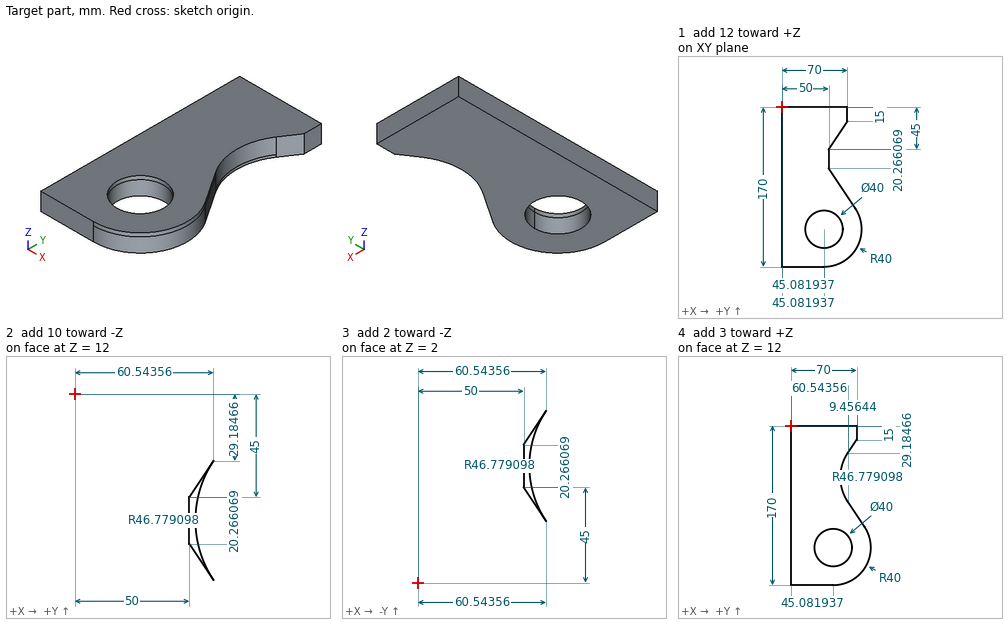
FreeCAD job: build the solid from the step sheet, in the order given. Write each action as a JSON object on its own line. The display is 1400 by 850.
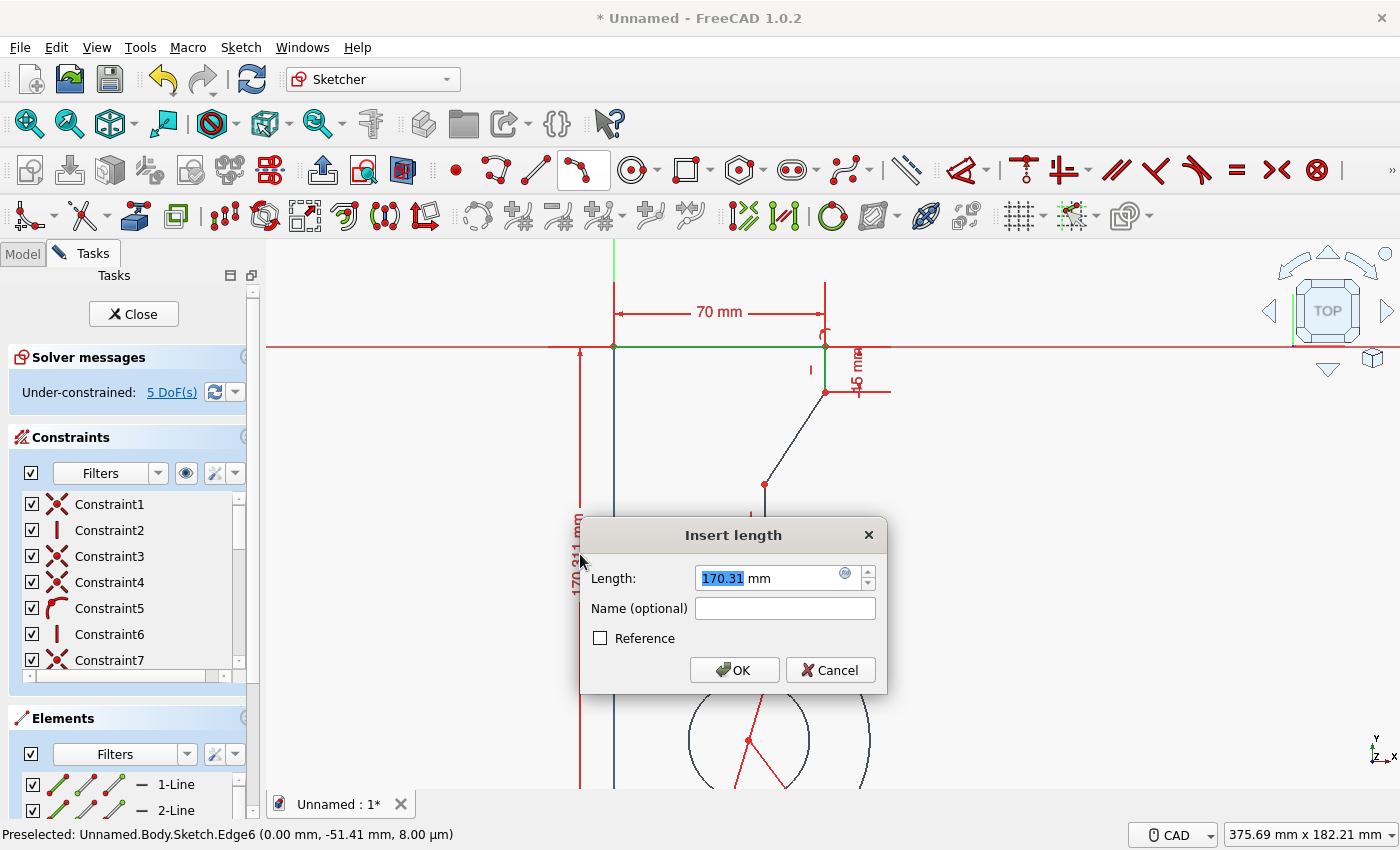
{"action": "type", "text": "170"}
{"action": "key", "text": "Return"}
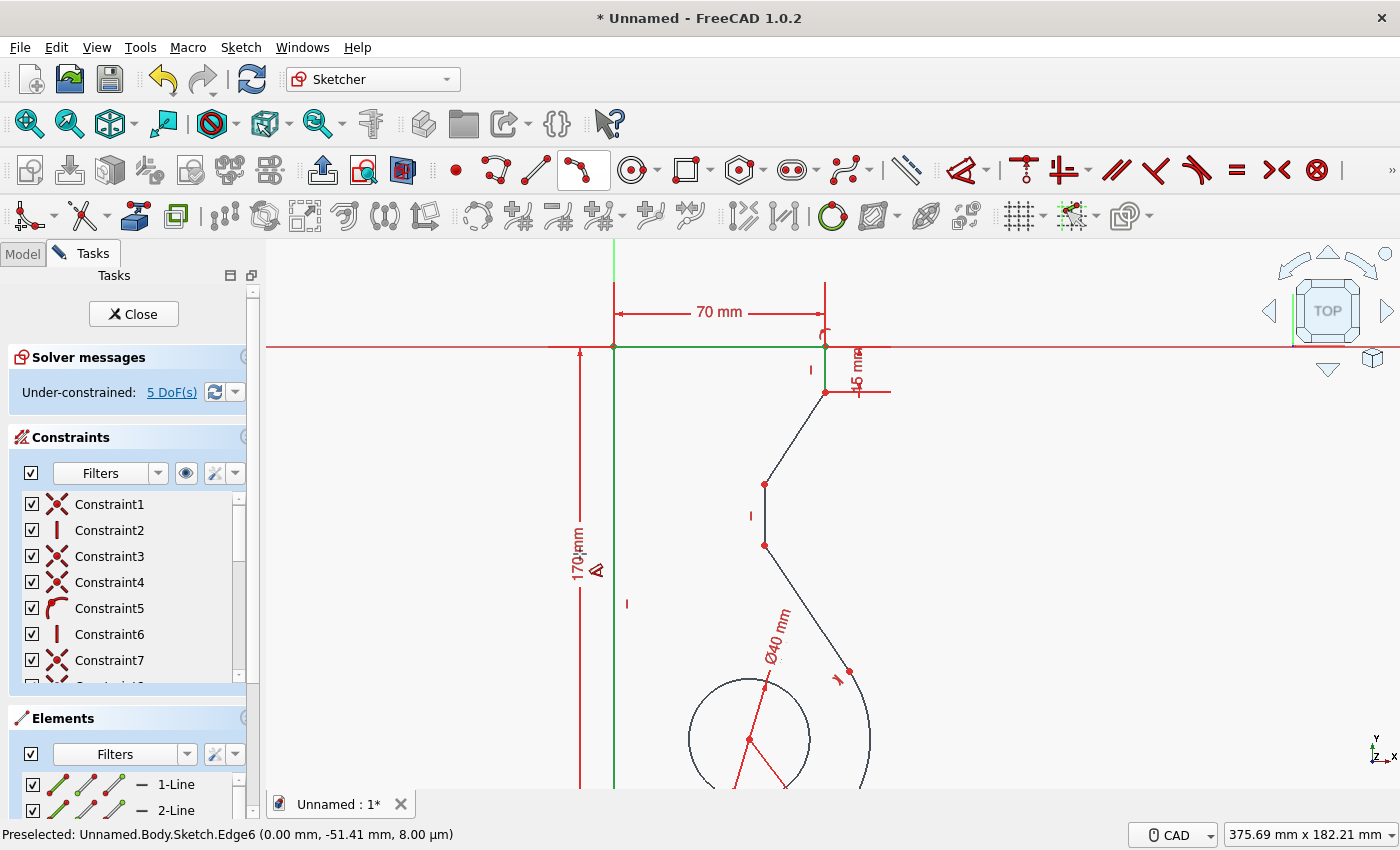
{"action": "left_click", "coordinate": [765, 546]}
{"action": "left_click", "coordinate": [636, 313]}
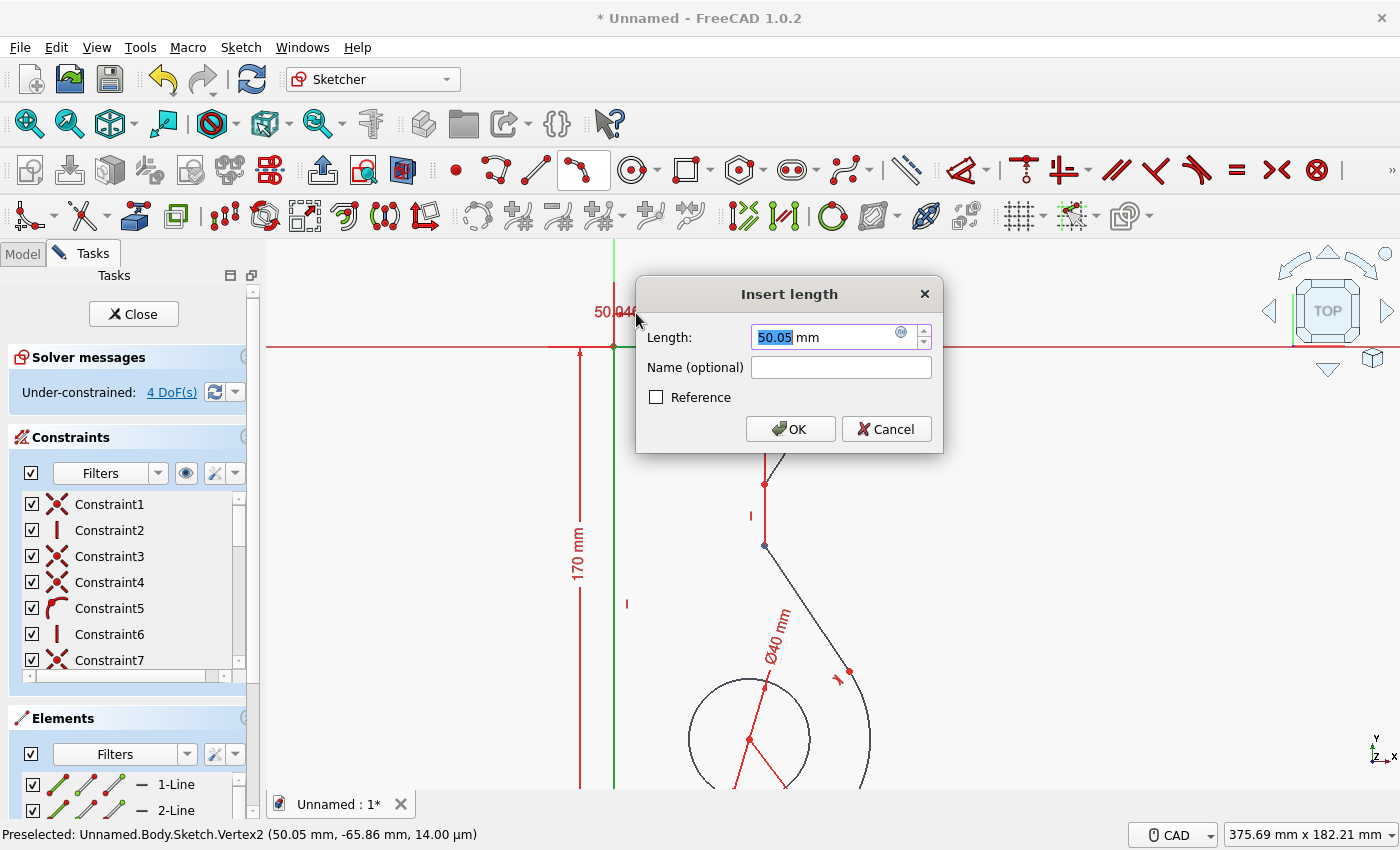
{"action": "type", "text": "50"}
{"action": "key", "text": "Return"}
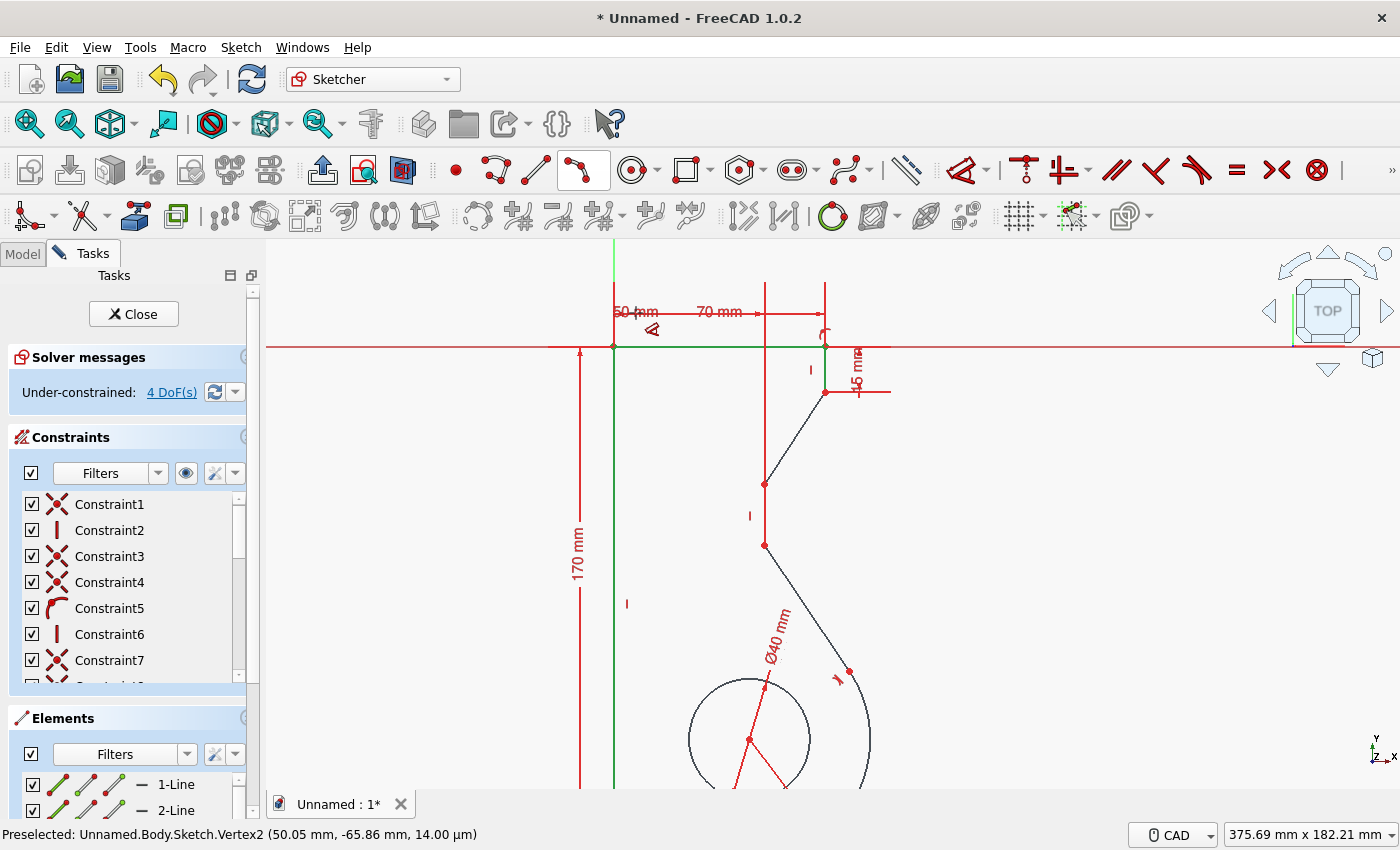
{"action": "left_click", "coordinate": [765, 485]}
{"action": "left_click", "coordinate": [580, 416]}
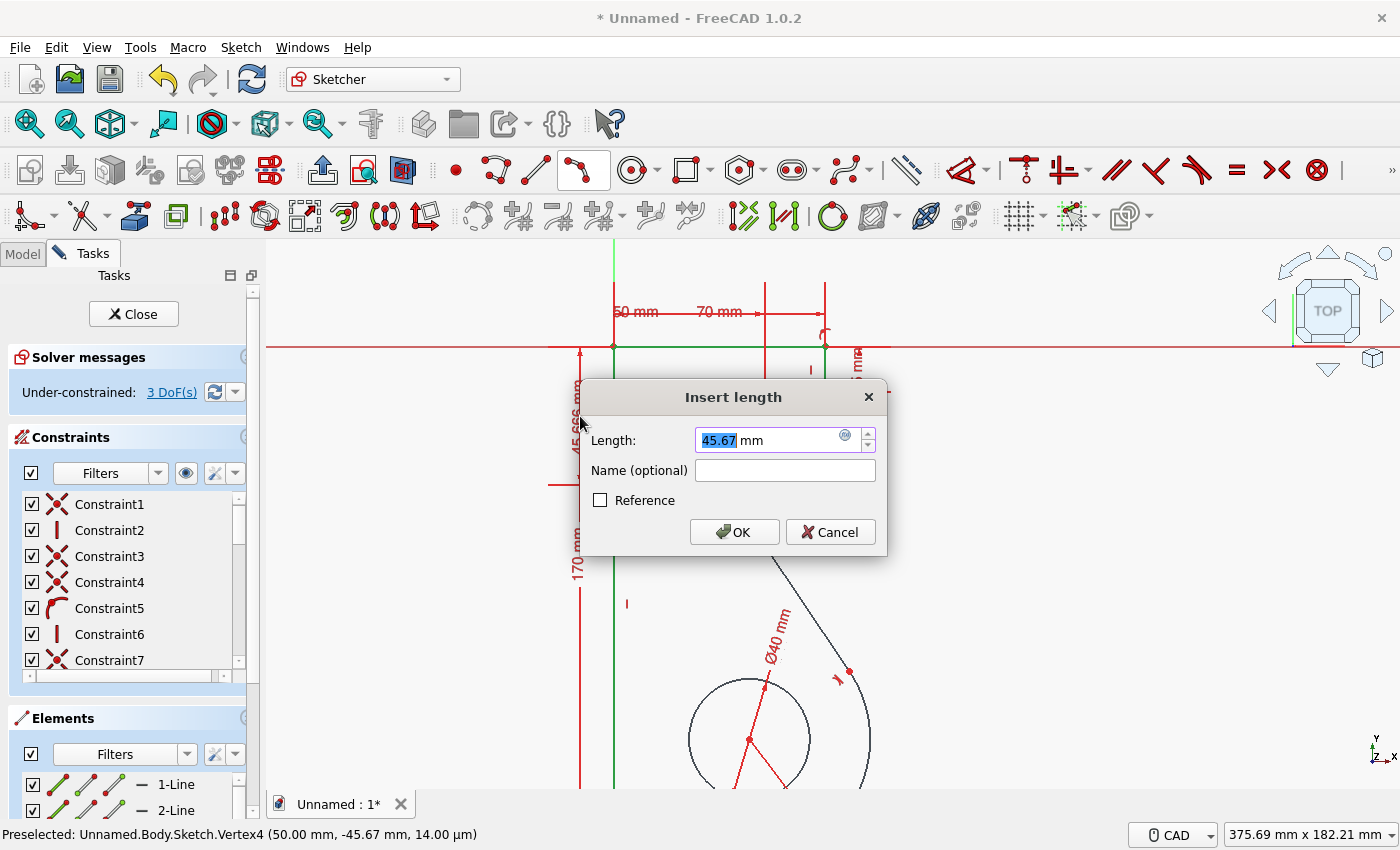
{"action": "type", "text": "45"}
{"action": "key", "text": "Return"}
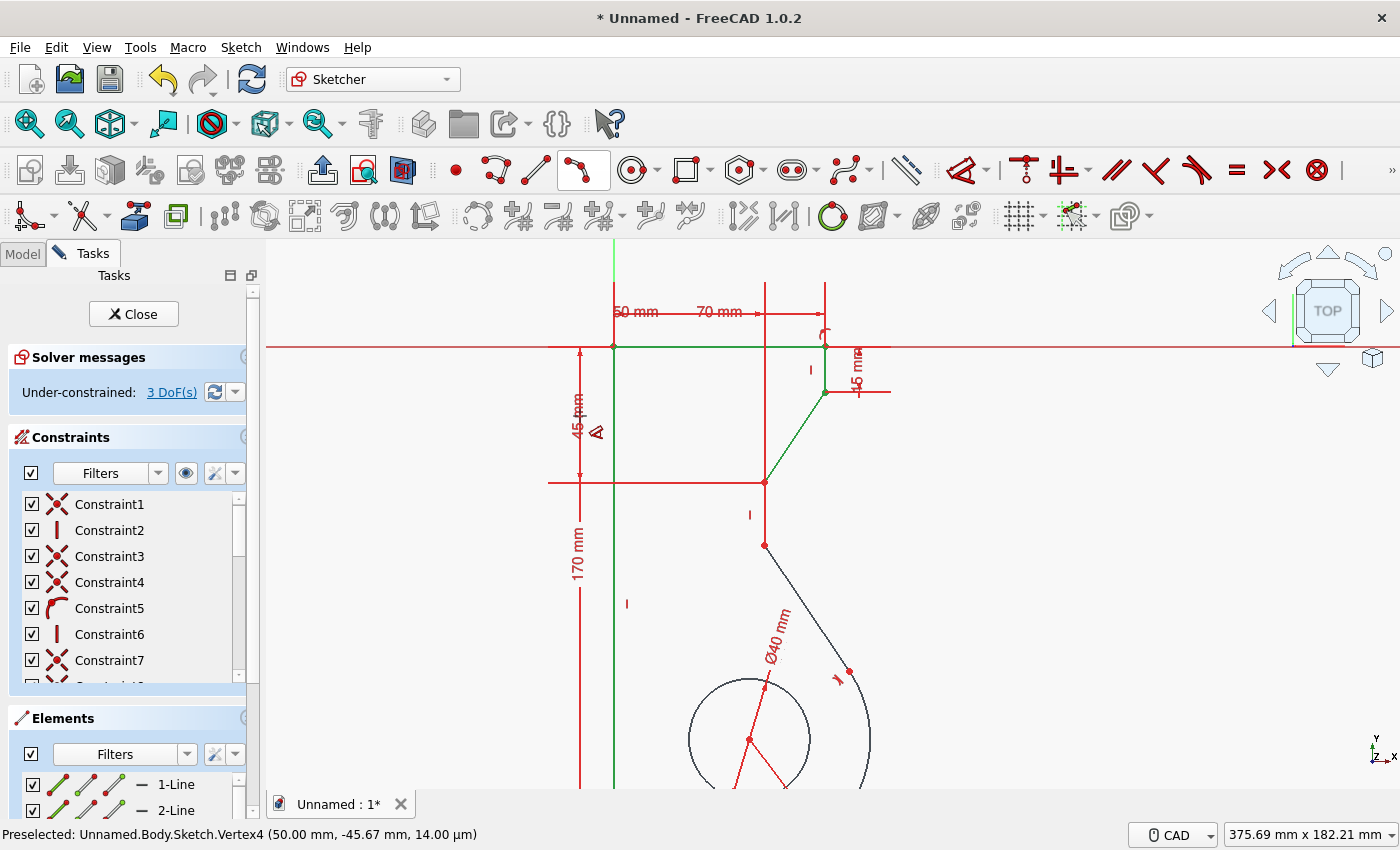
{"action": "left_click", "coordinate": [765, 527]}
{"action": "left_click", "coordinate": [799, 514]}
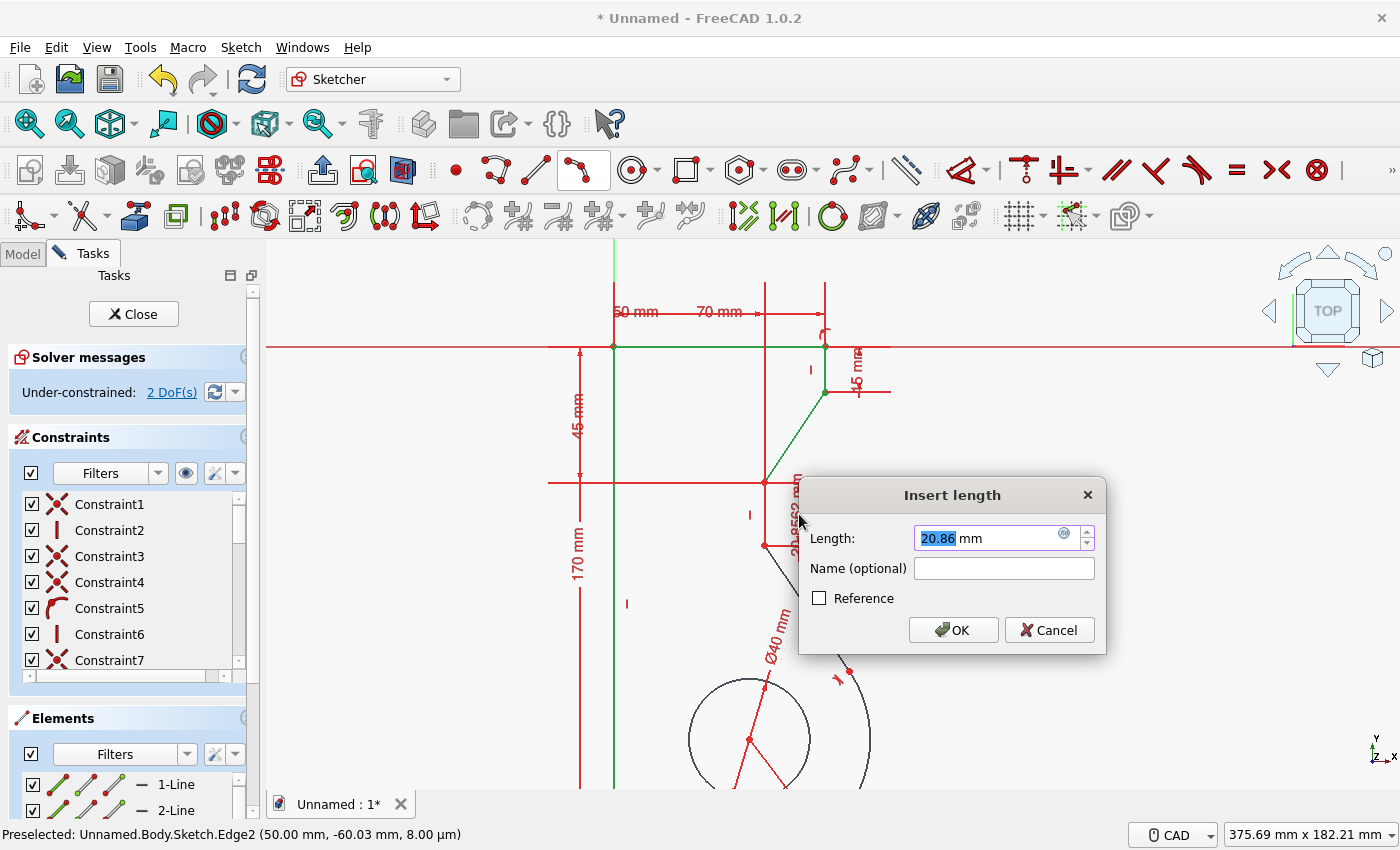
{"action": "type", "text": "20.266069"}
{"action": "key", "text": "Return"}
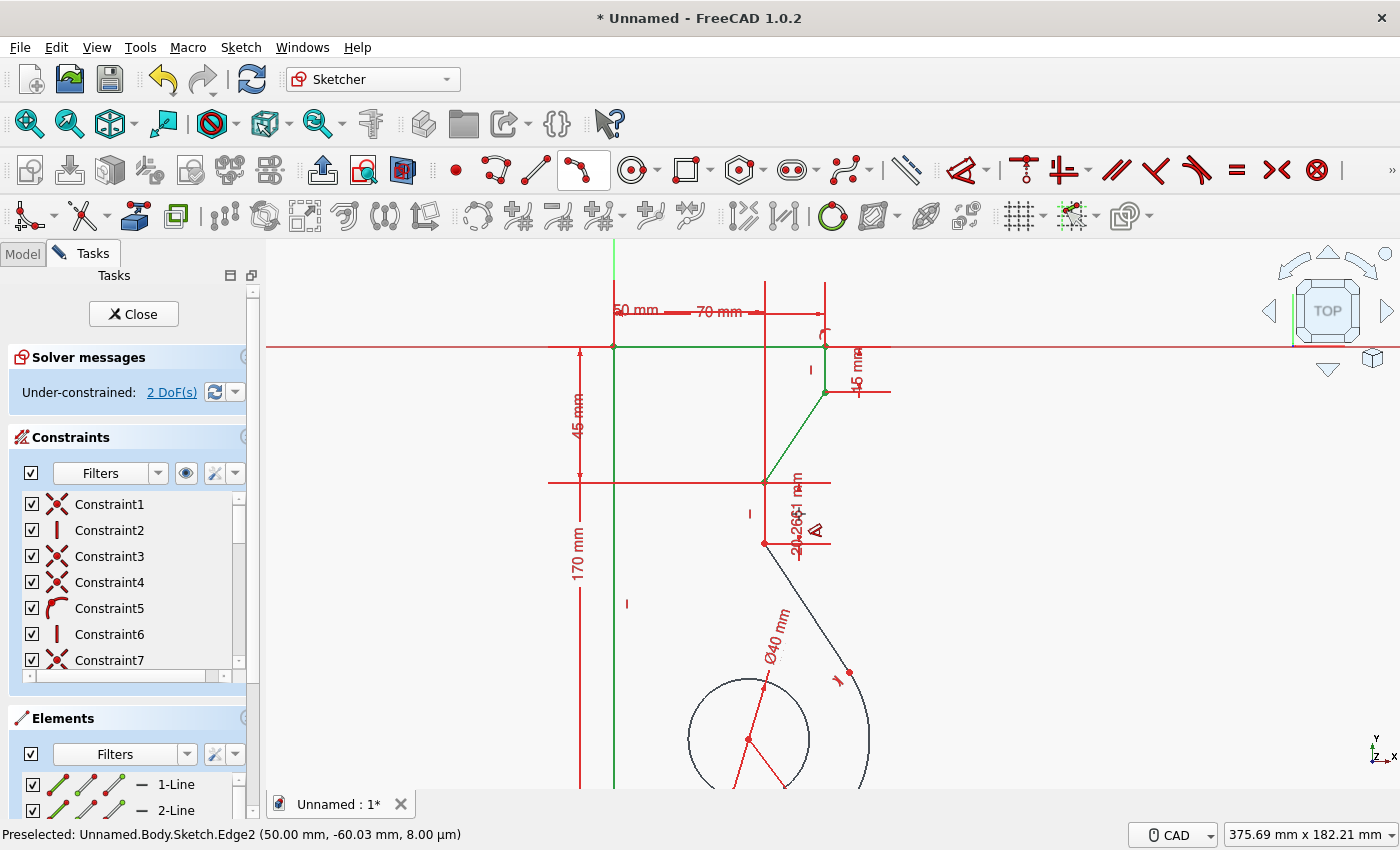
{"action": "scroll", "coordinate": [824, 332], "scroll_direction": "down", "scroll_amount": 2}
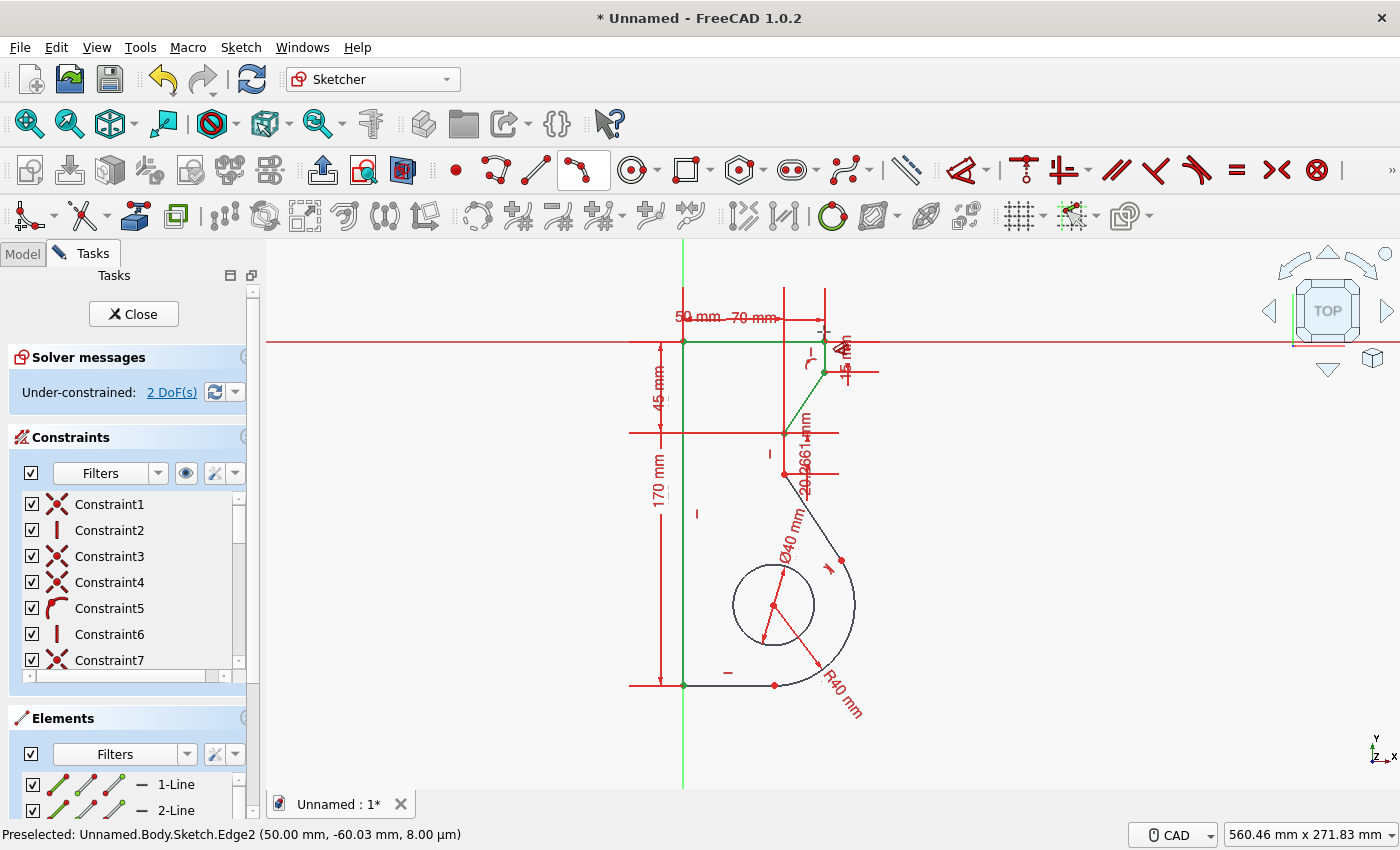
{"action": "left_click", "coordinate": [711, 686]}
{"action": "left_click", "coordinate": [729, 720]}